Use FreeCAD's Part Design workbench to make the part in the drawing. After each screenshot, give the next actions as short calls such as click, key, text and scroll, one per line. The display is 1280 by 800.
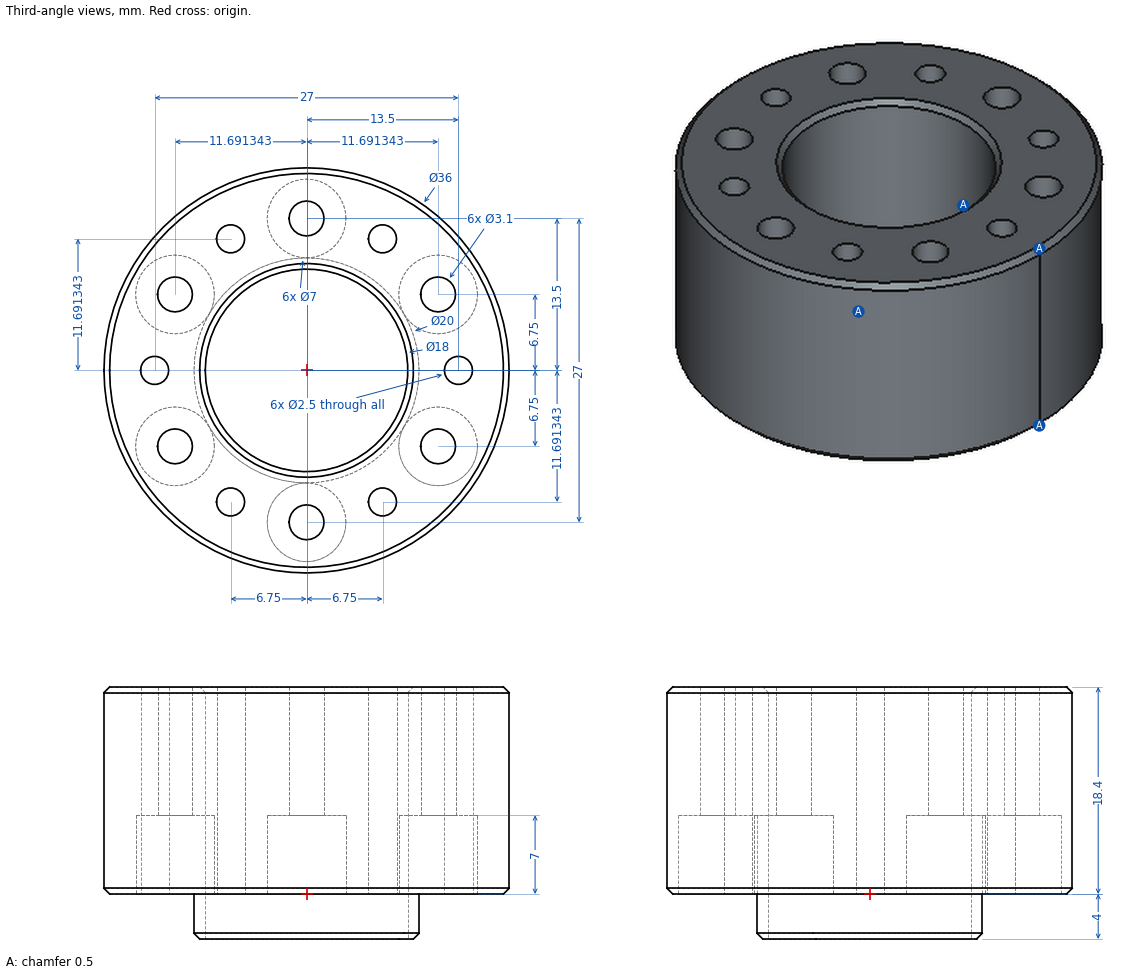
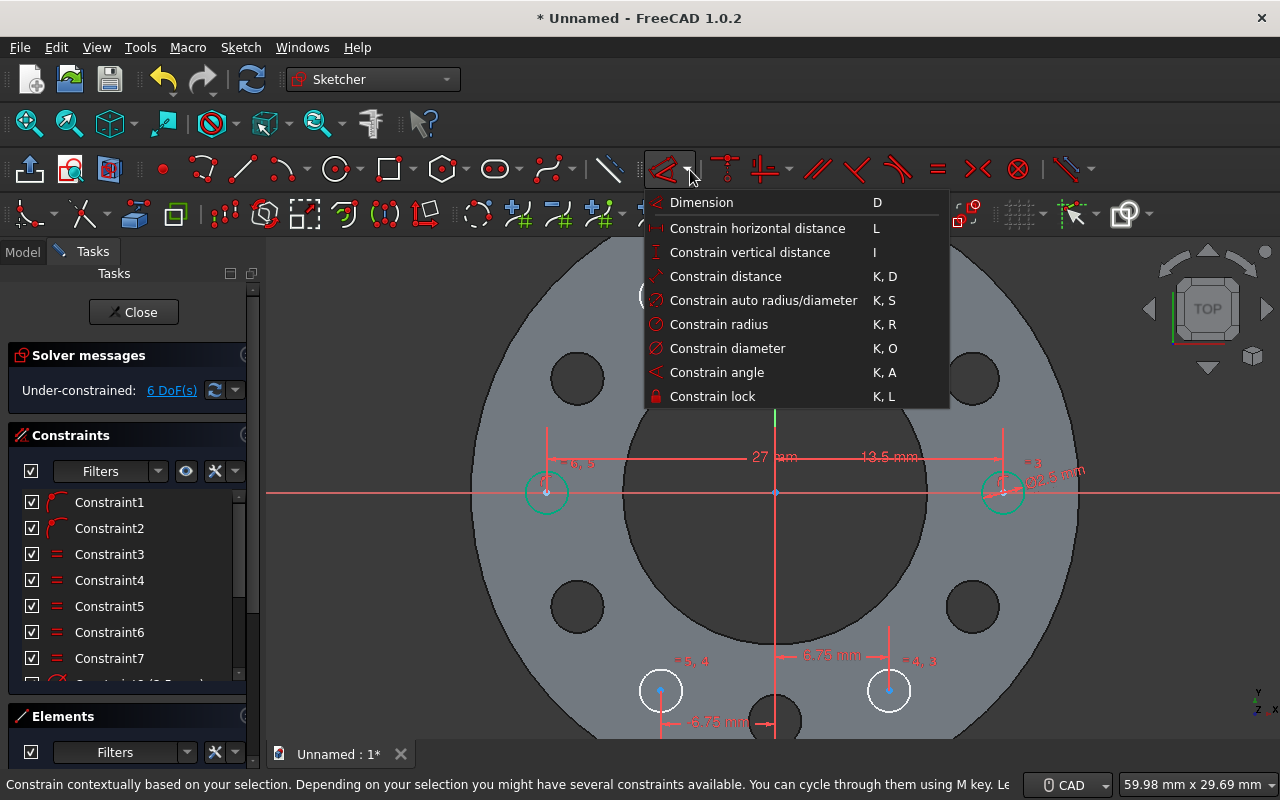
click(797, 228)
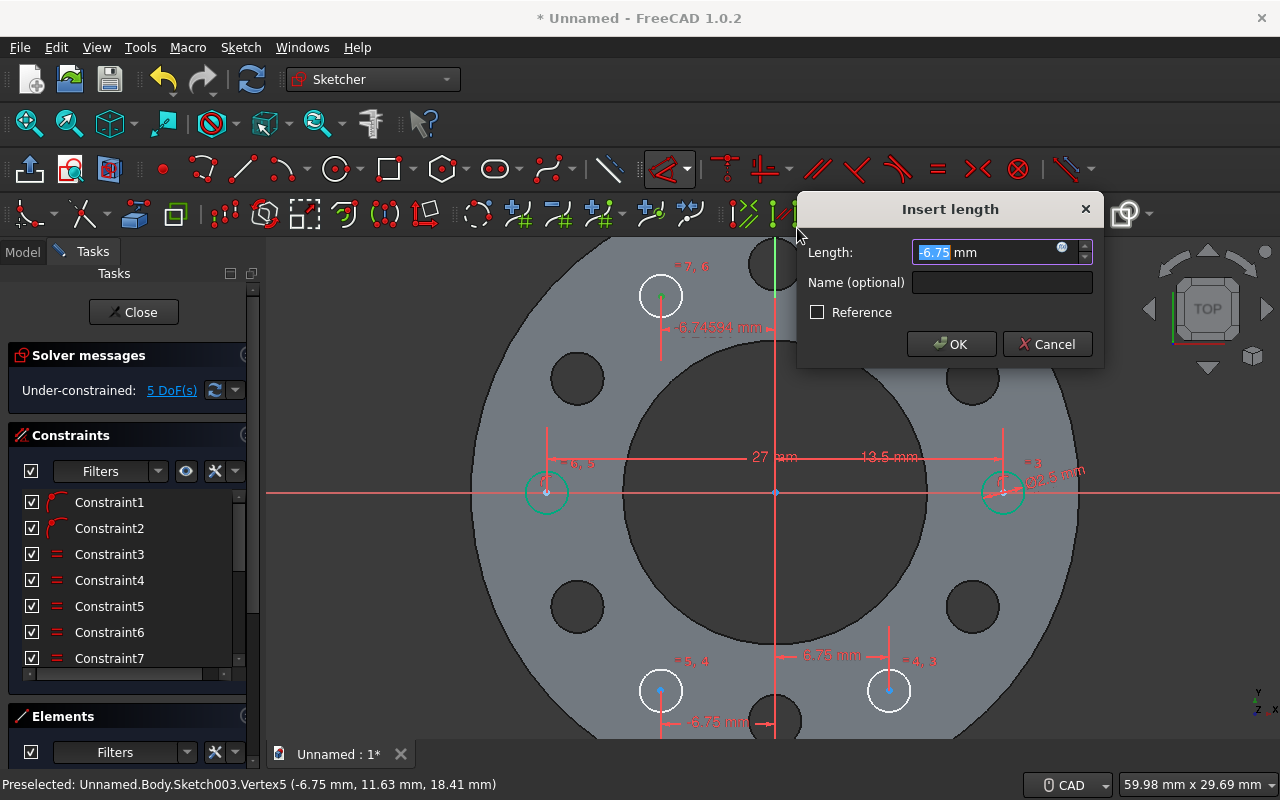
text(-6.75)
key(Return)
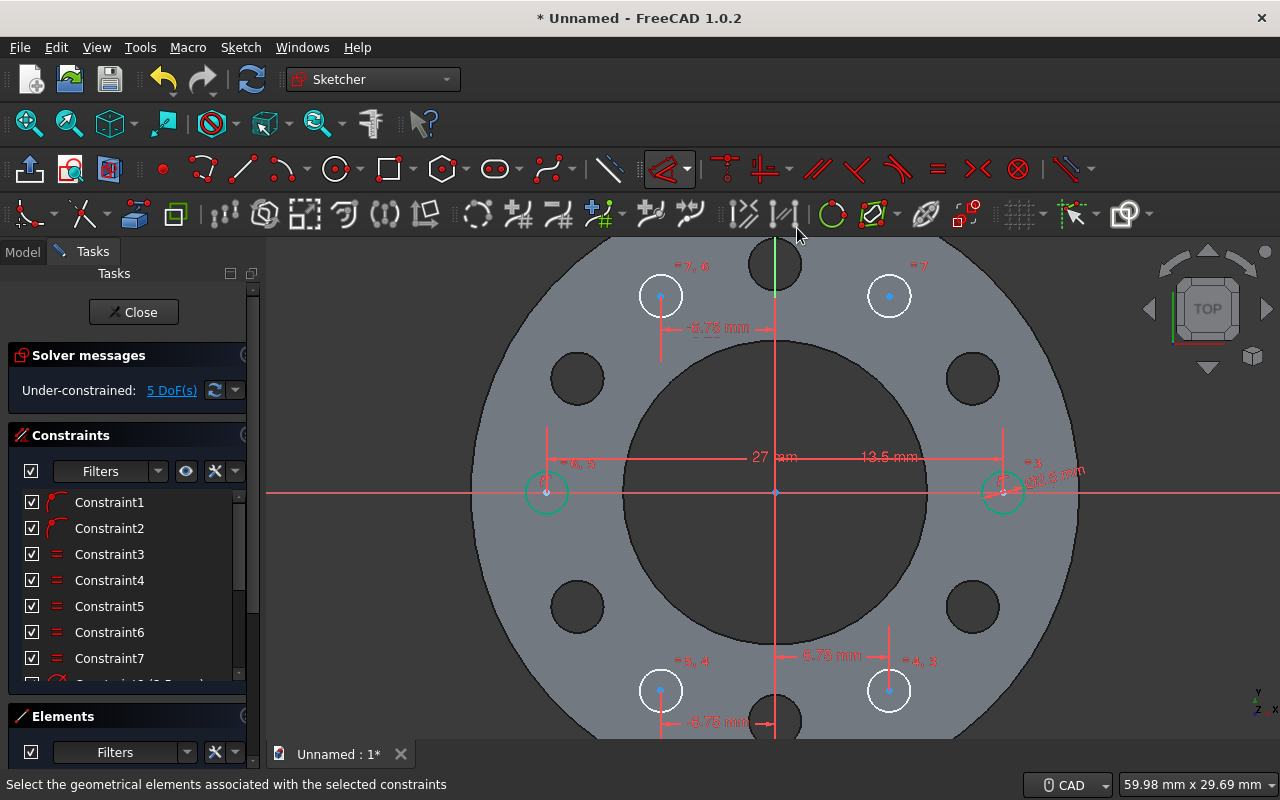
click(889, 296)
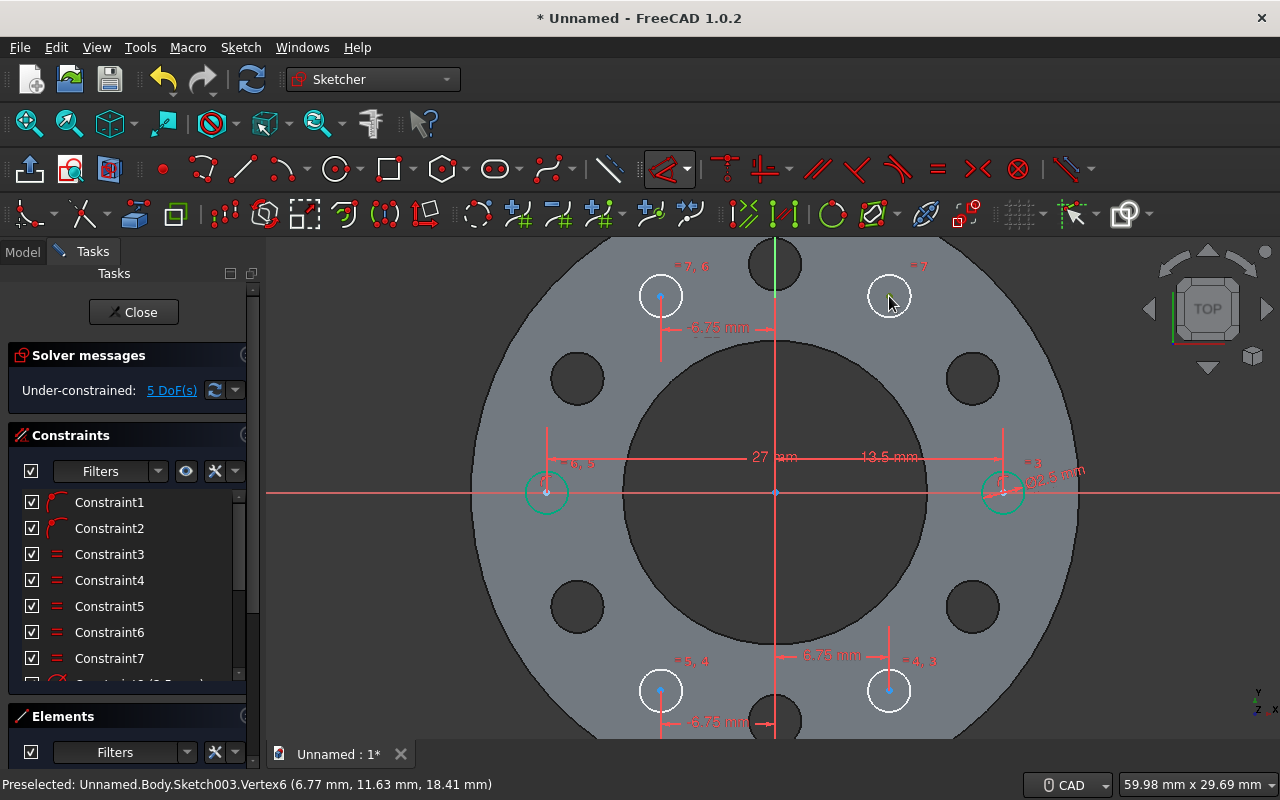
key(l)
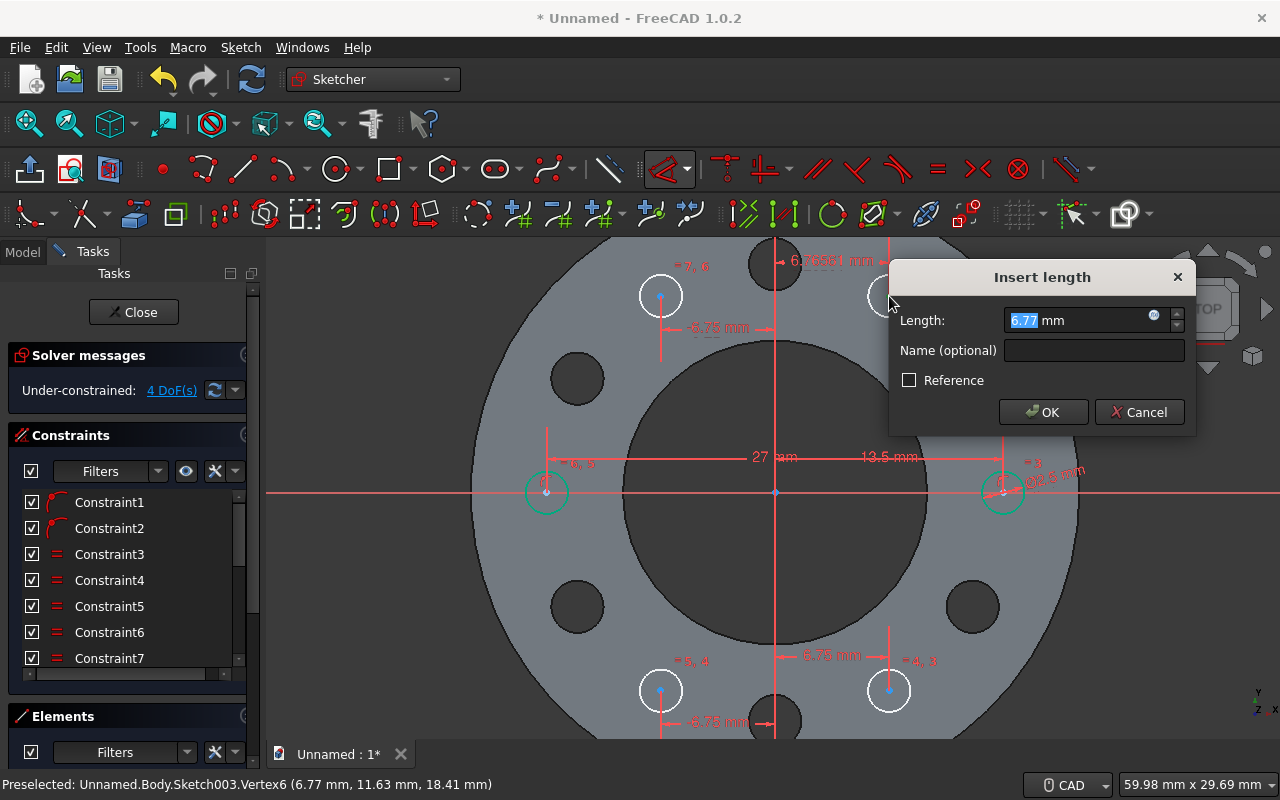
text(6.75)
key(Return)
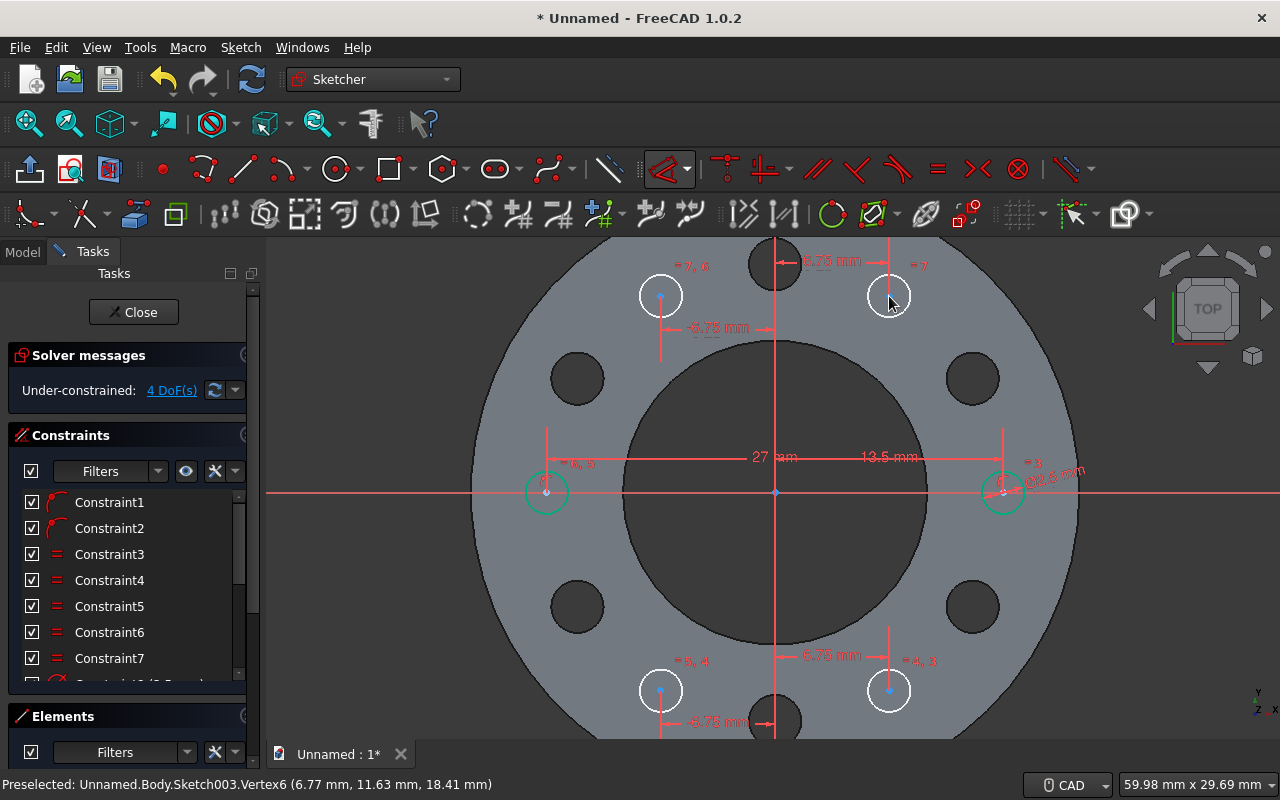
click(889, 691)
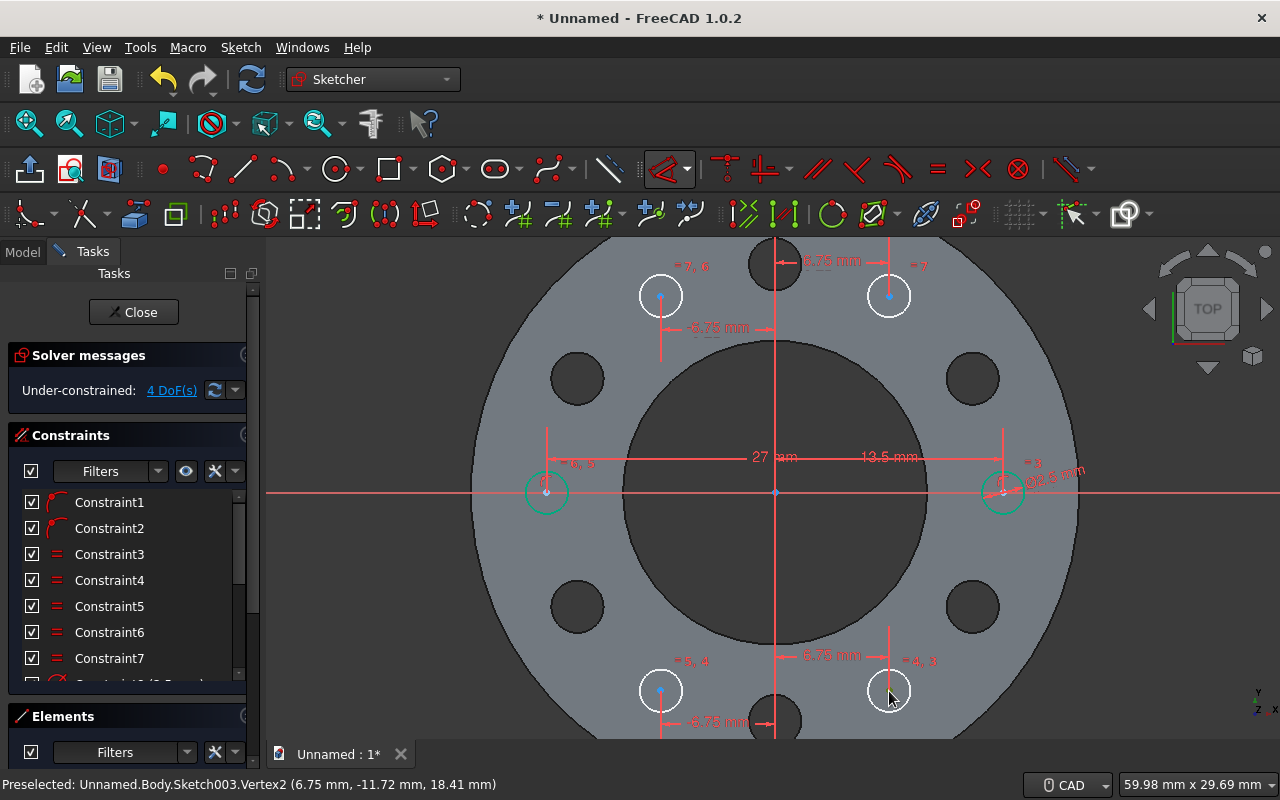
key(i)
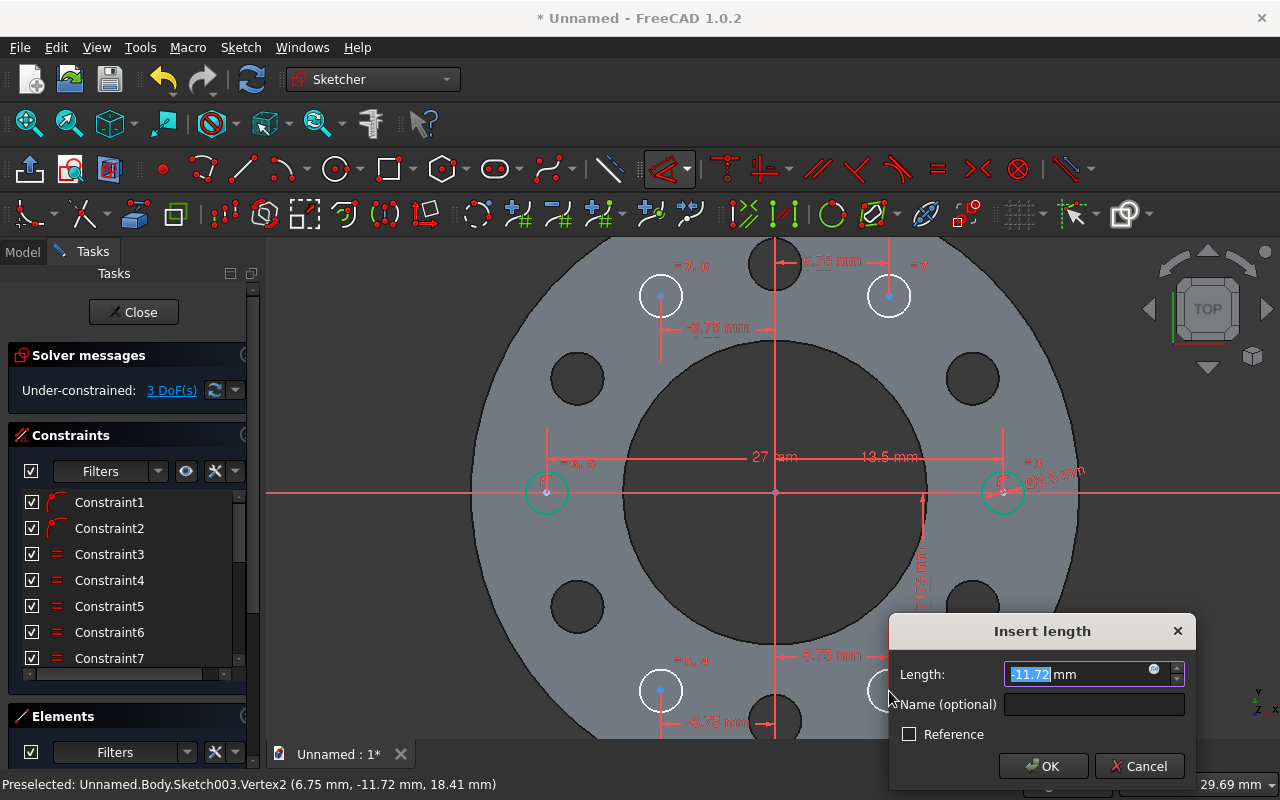
text(-11.691343)
key(Return)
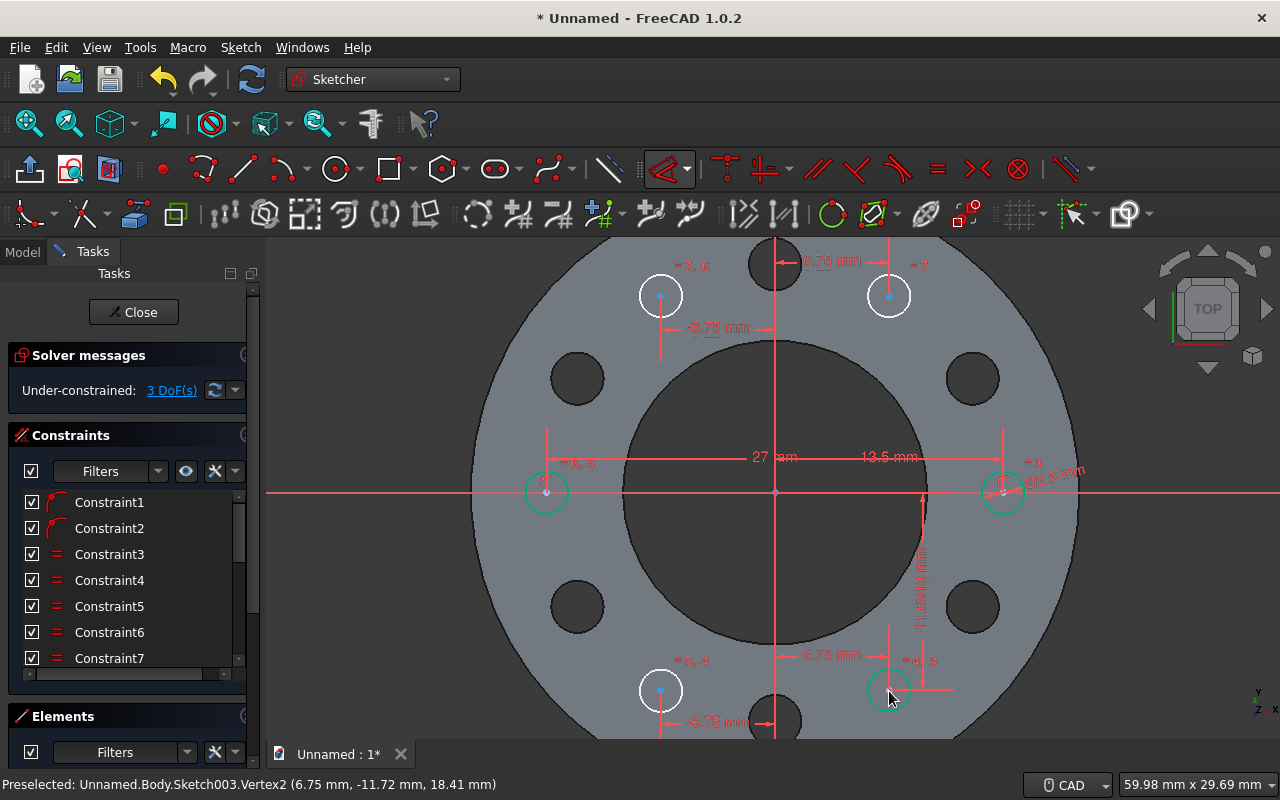
click(661, 691)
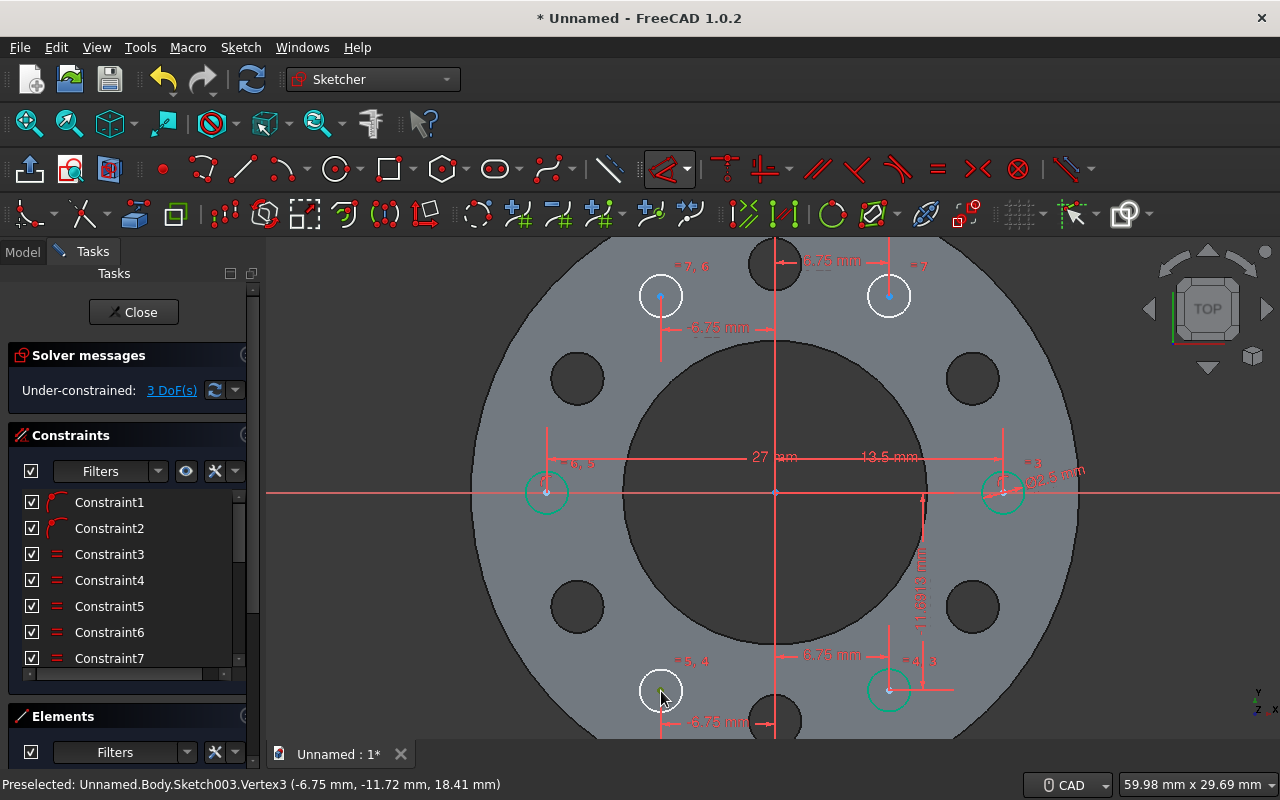
key(i)